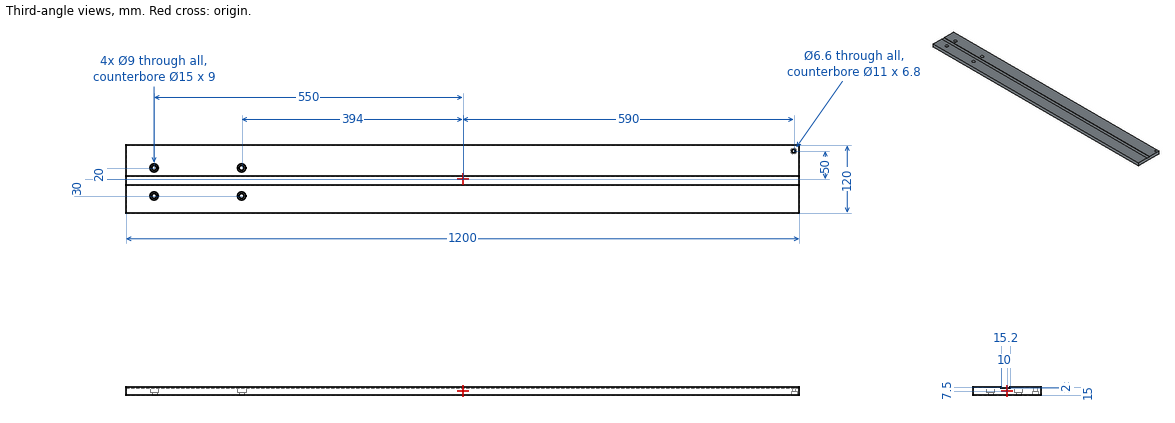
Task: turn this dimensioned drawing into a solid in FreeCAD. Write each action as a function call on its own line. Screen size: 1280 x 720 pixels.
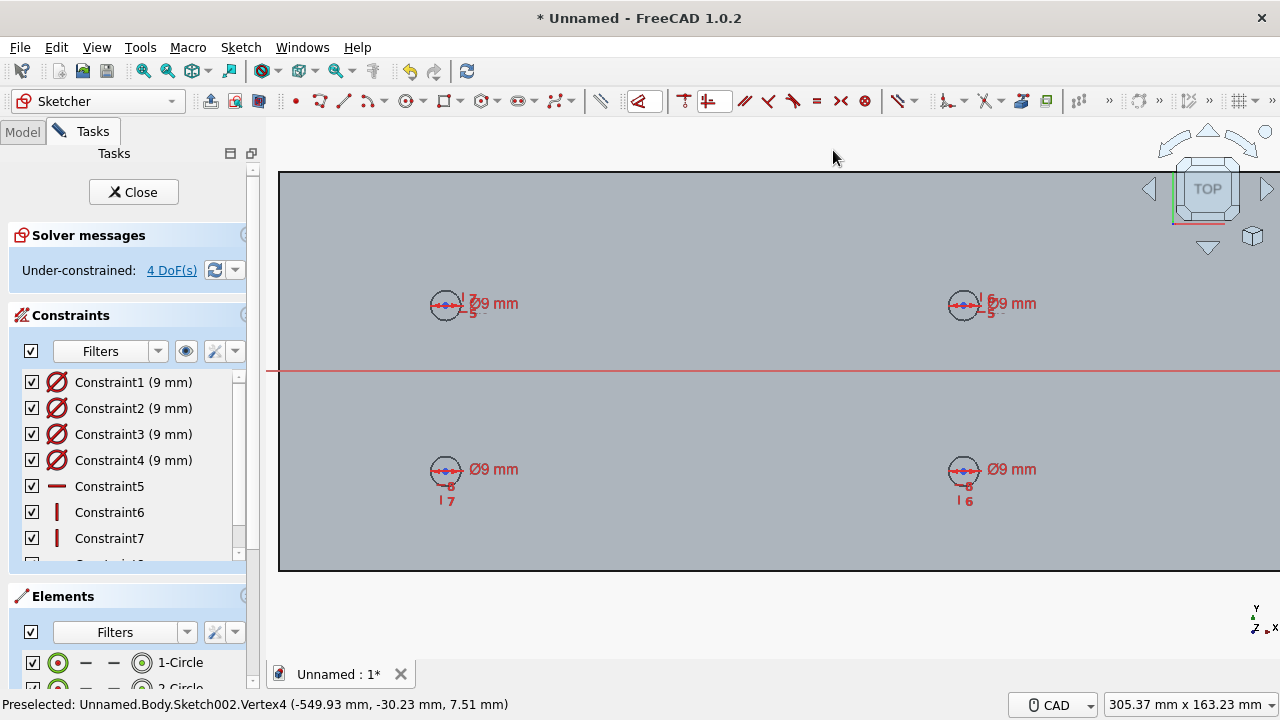
click(446, 306)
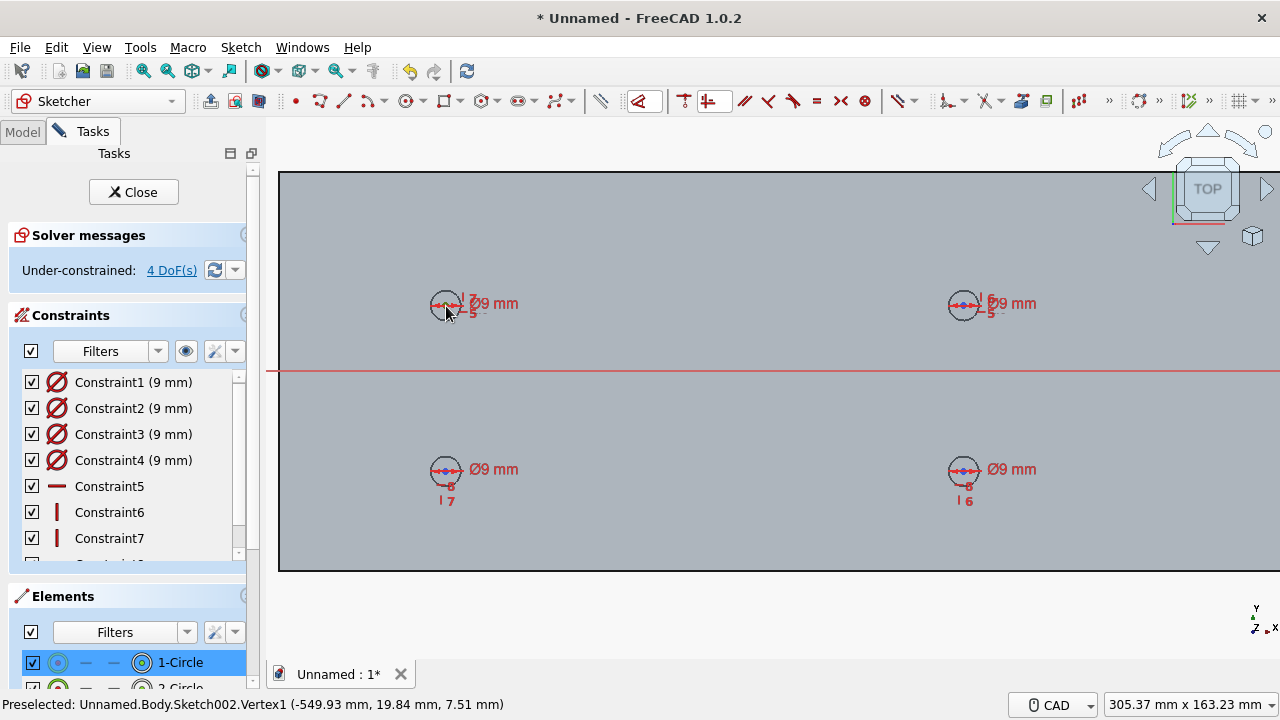
key(i)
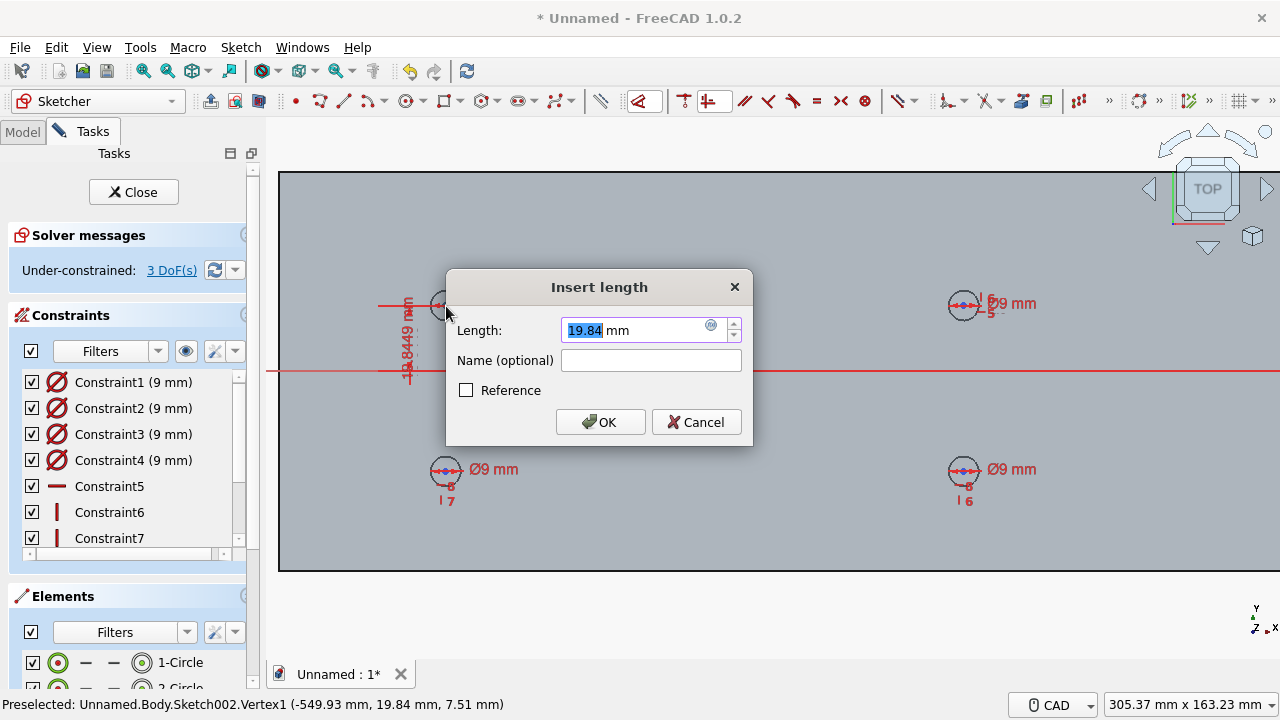
text(20)
key(Return)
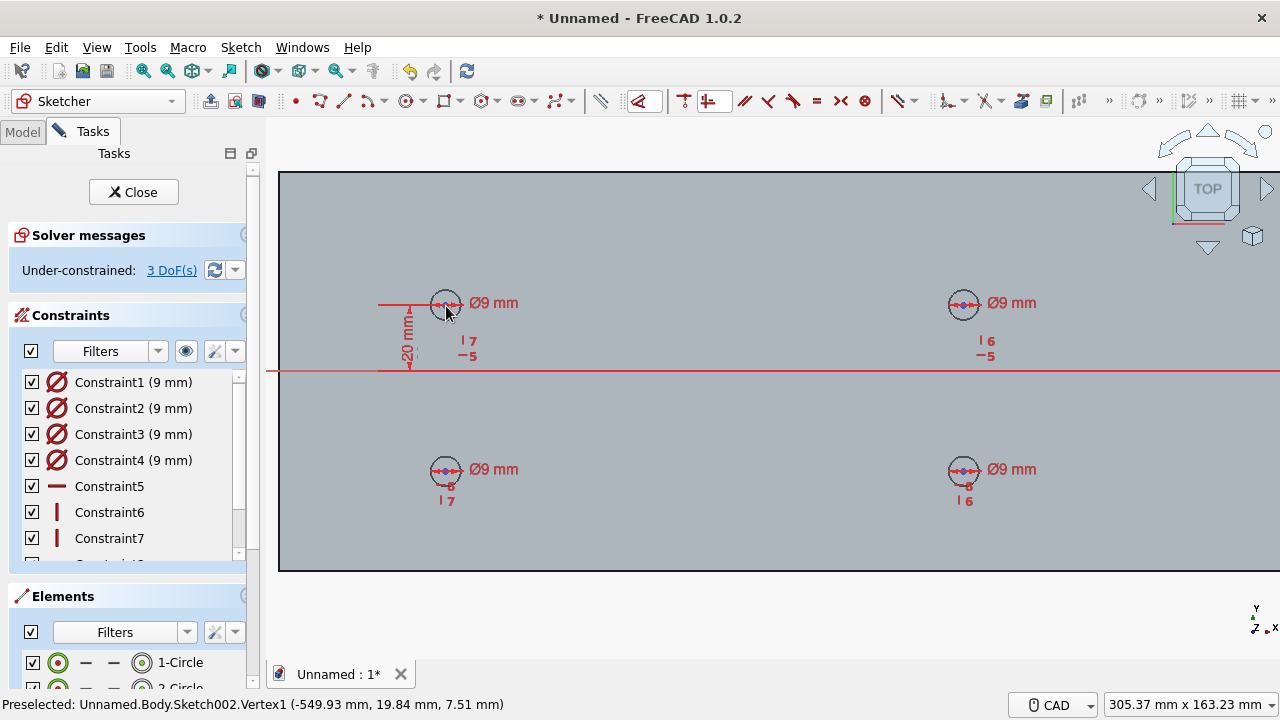
click(964, 471)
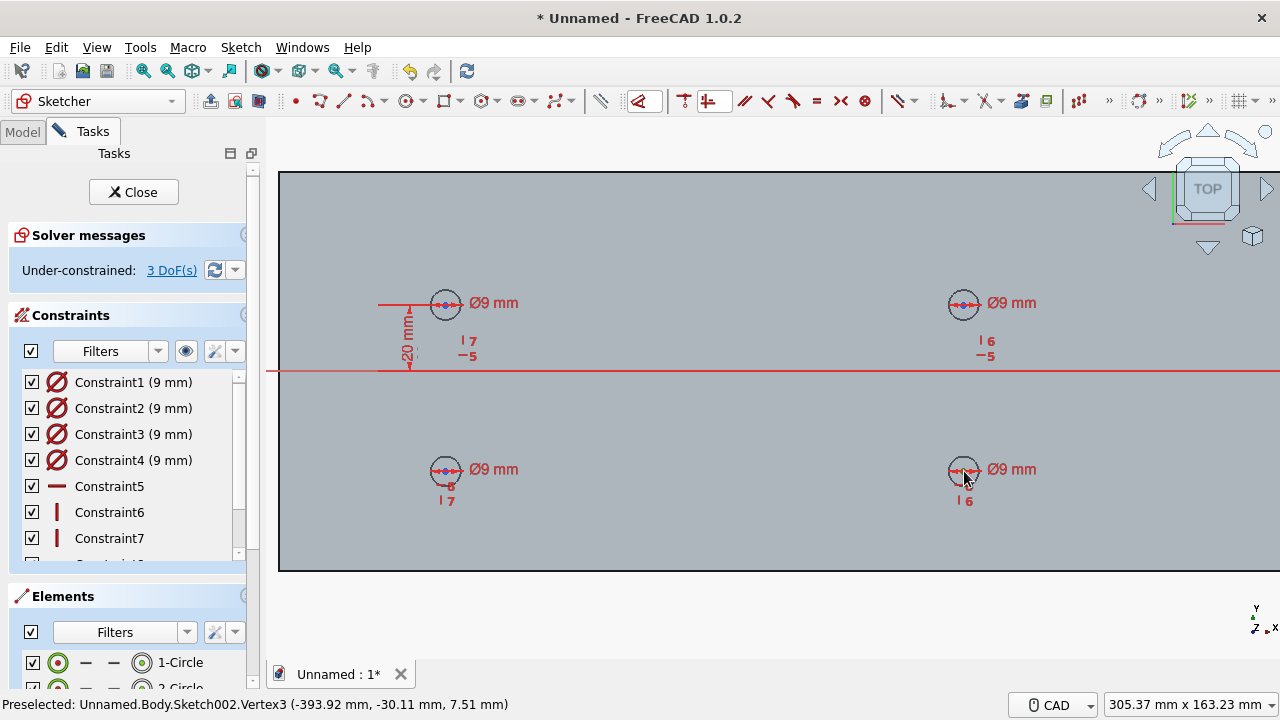
click(656, 102)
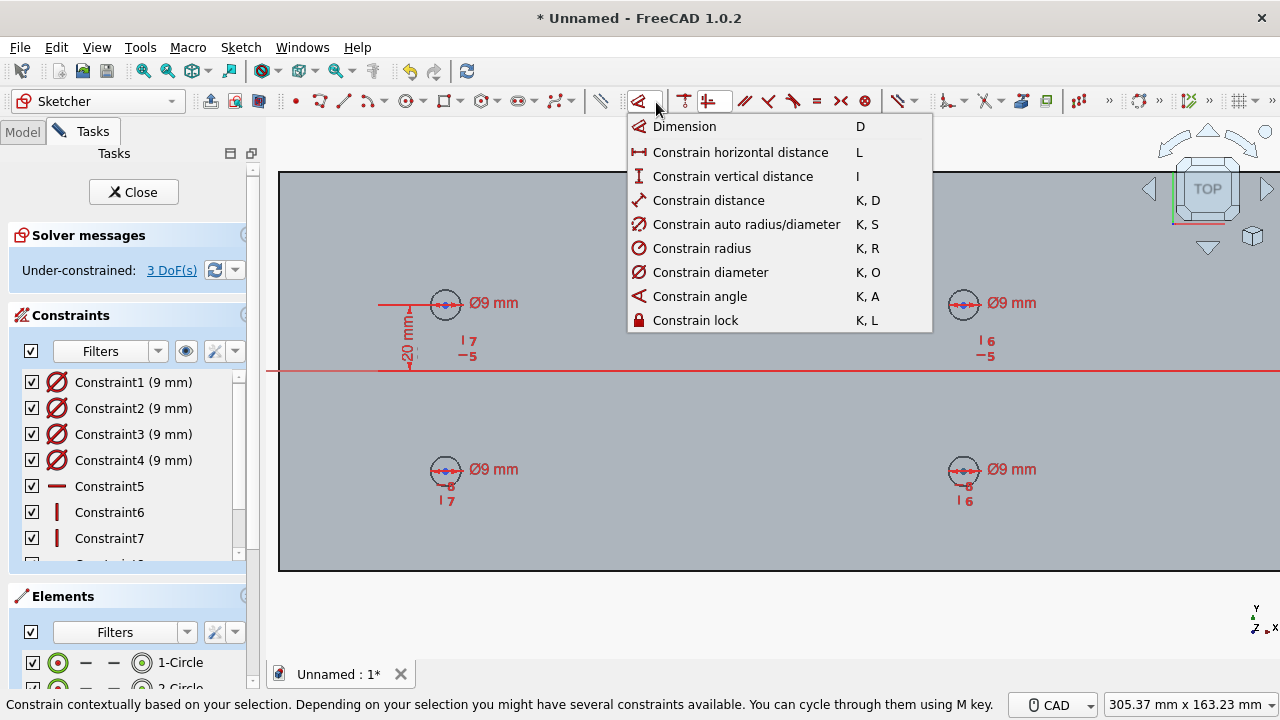
click(780, 176)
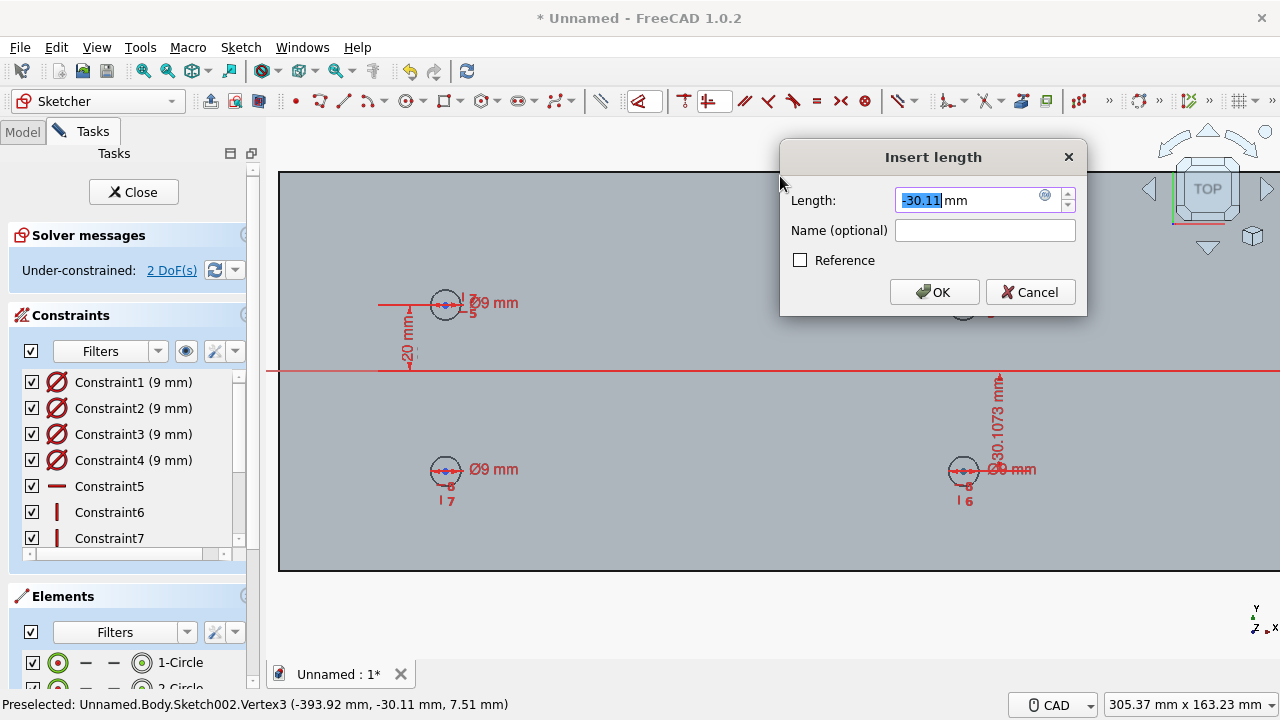
text(-30)
key(Return)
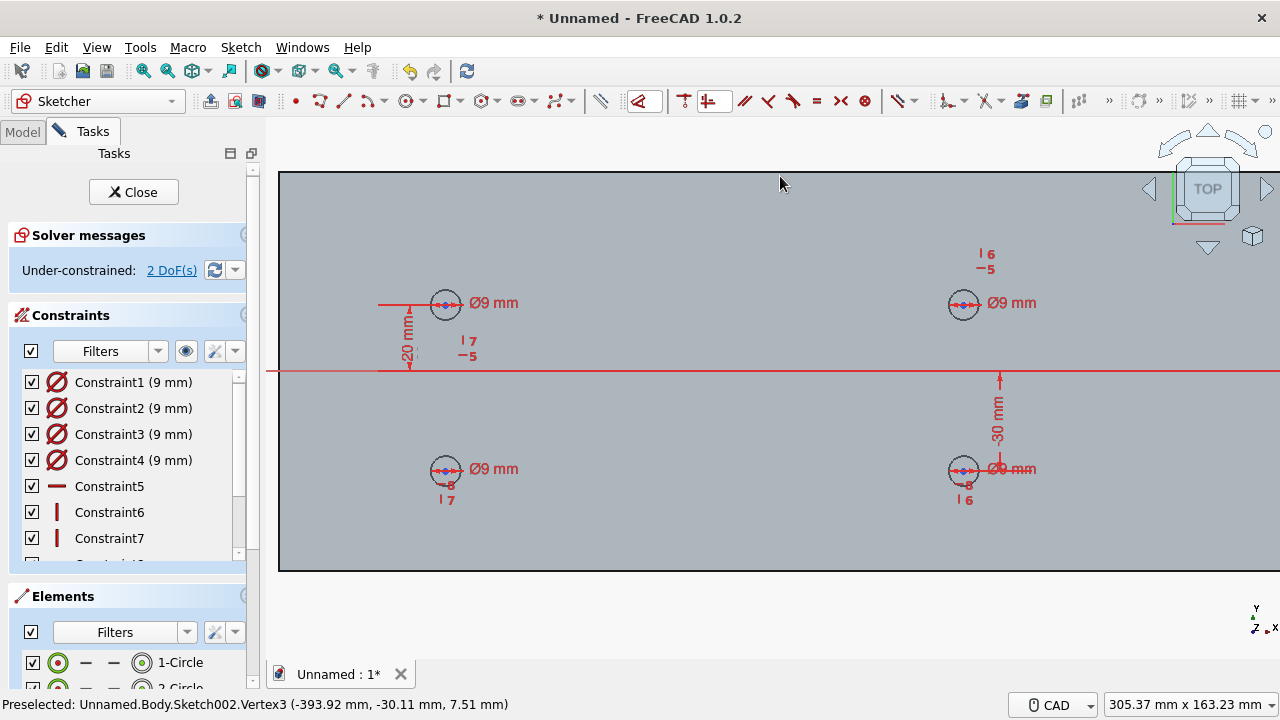
click(446, 305)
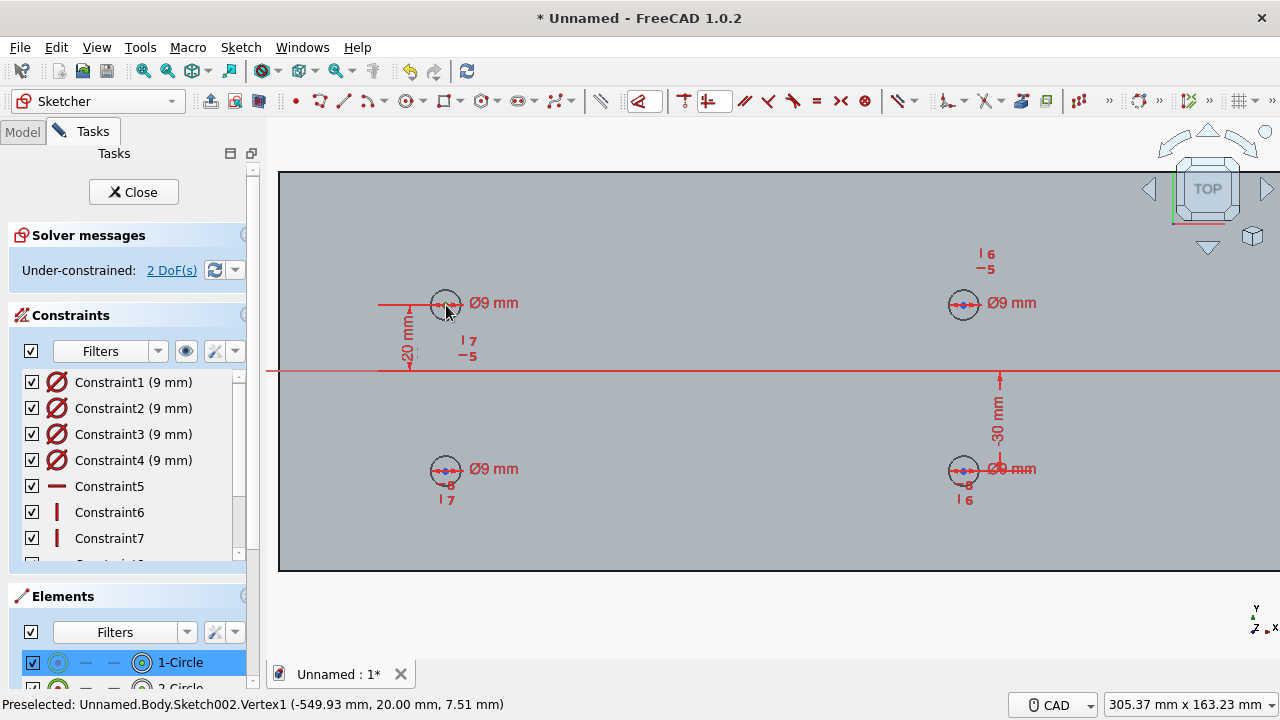
click(656, 102)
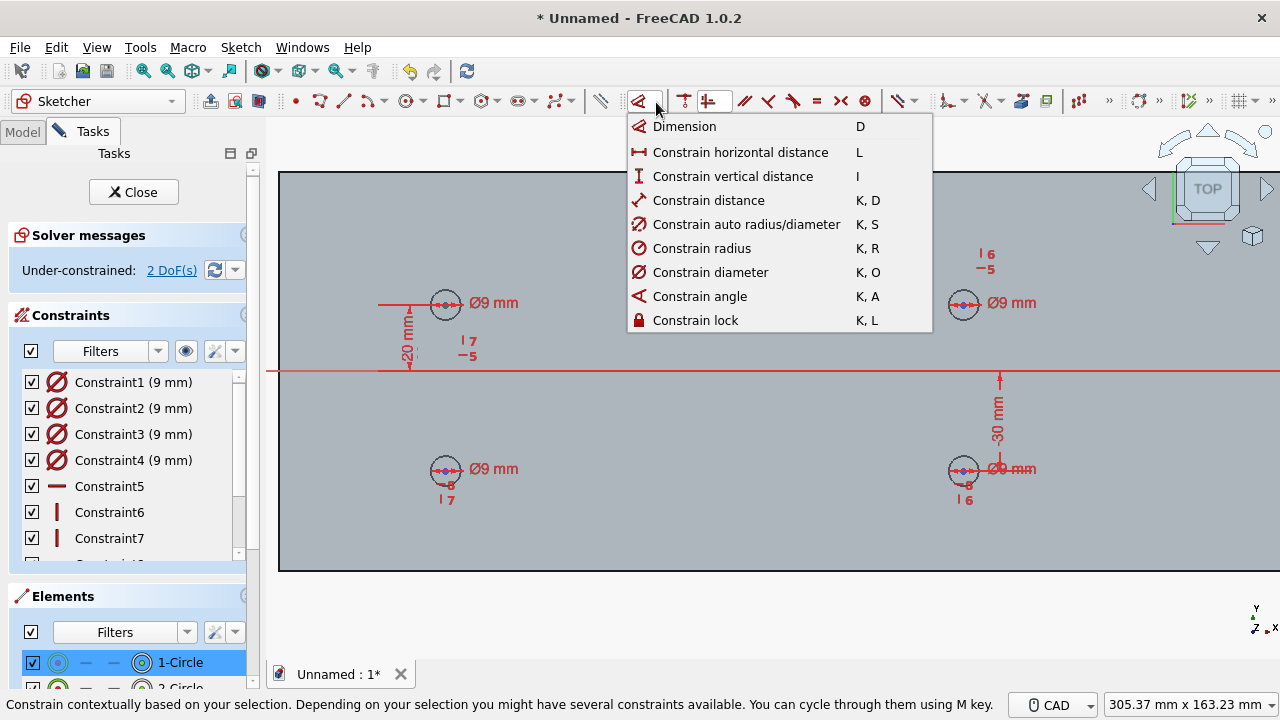
click(780, 152)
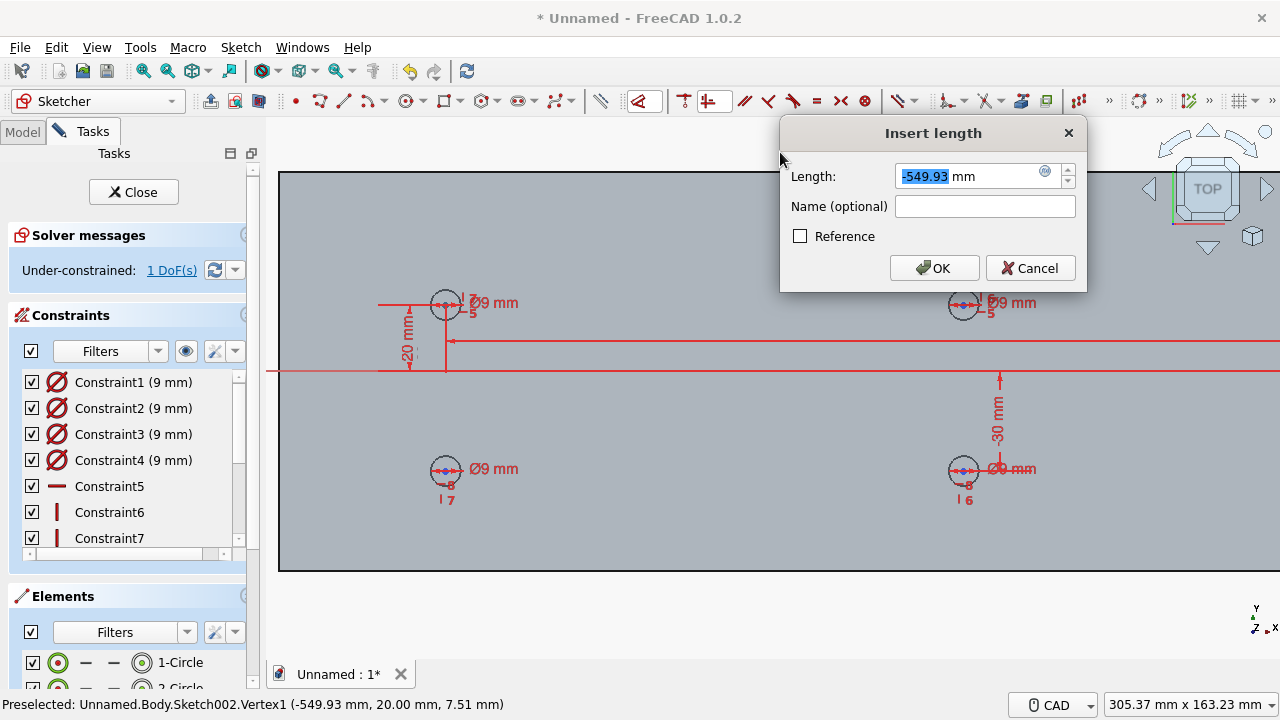
text(-550)
key(Return)